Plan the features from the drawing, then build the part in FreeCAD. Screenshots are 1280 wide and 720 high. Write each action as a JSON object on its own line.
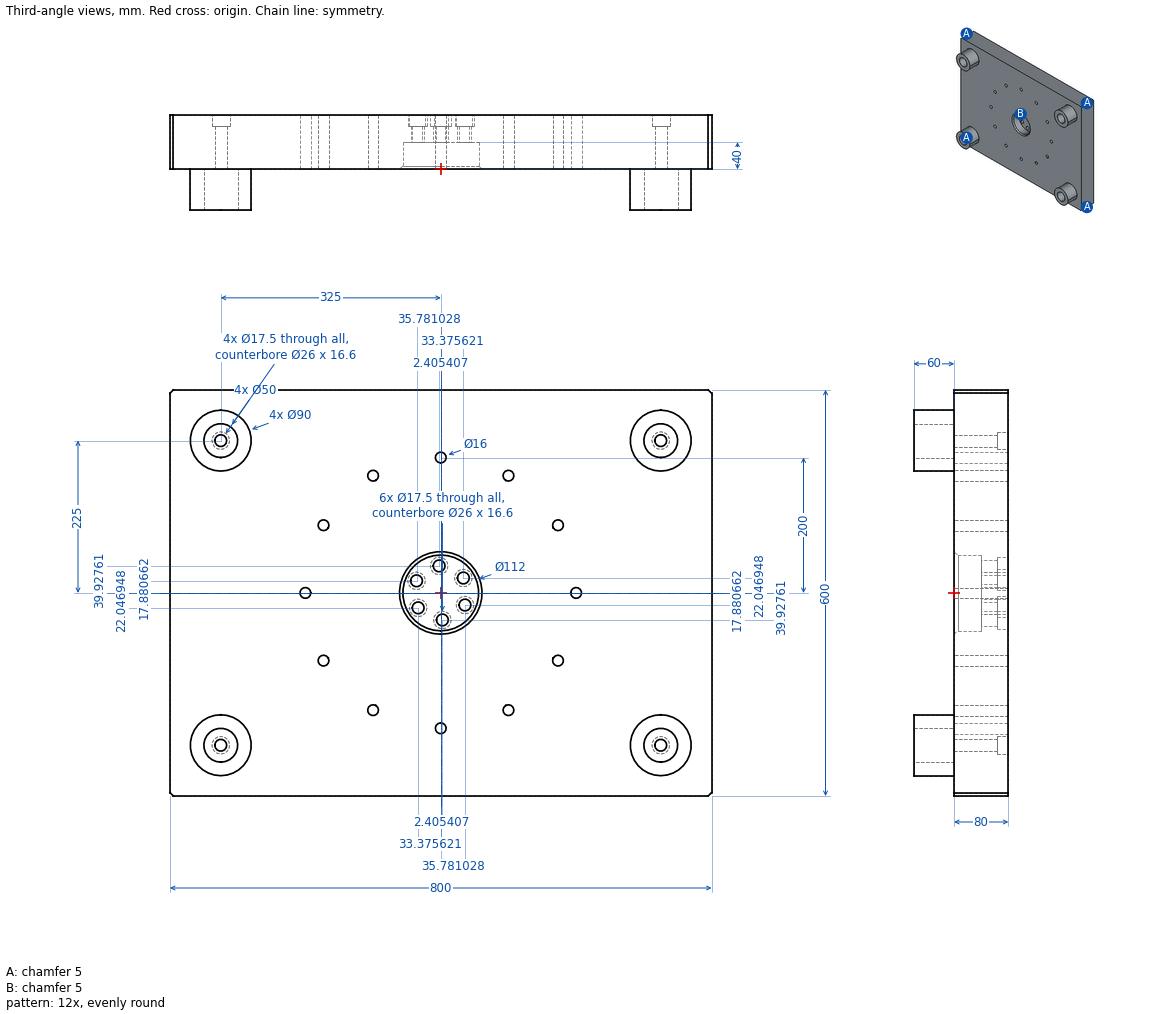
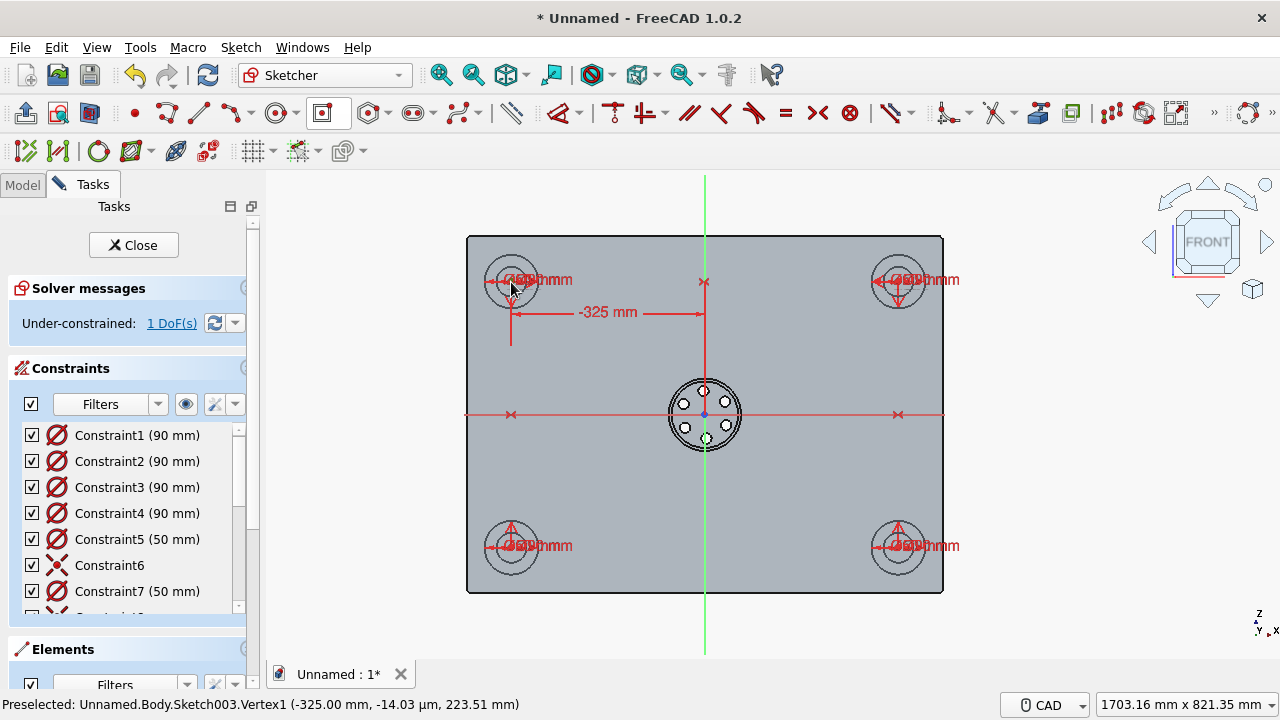
{"action": "key", "text": "i"}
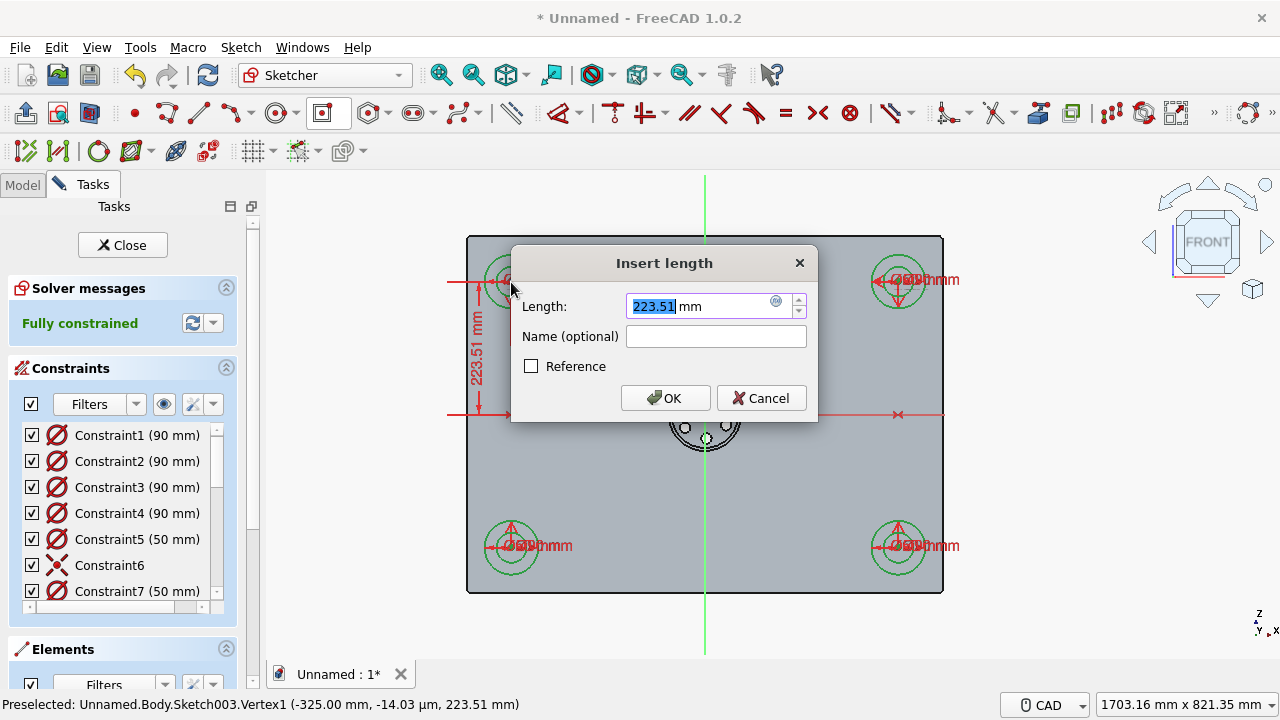
{"action": "type", "text": "225"}
{"action": "key", "text": "Return"}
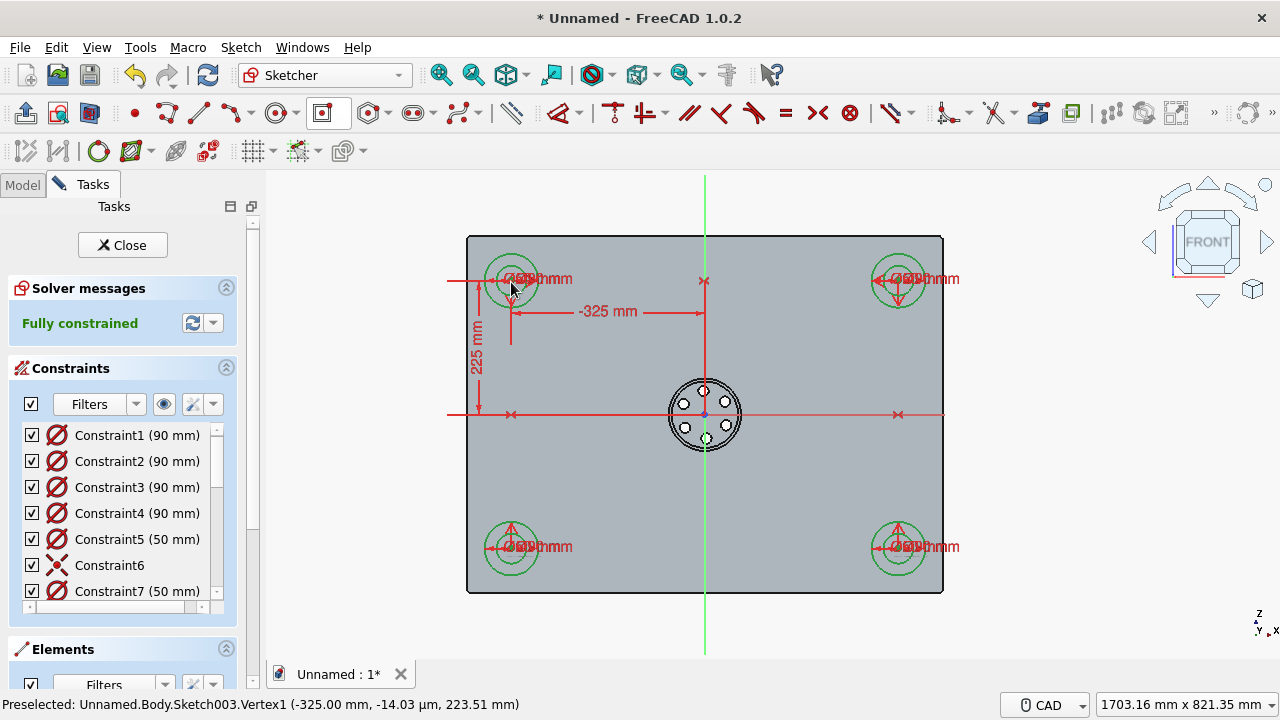
{"action": "left_click", "coordinate": [123, 245]}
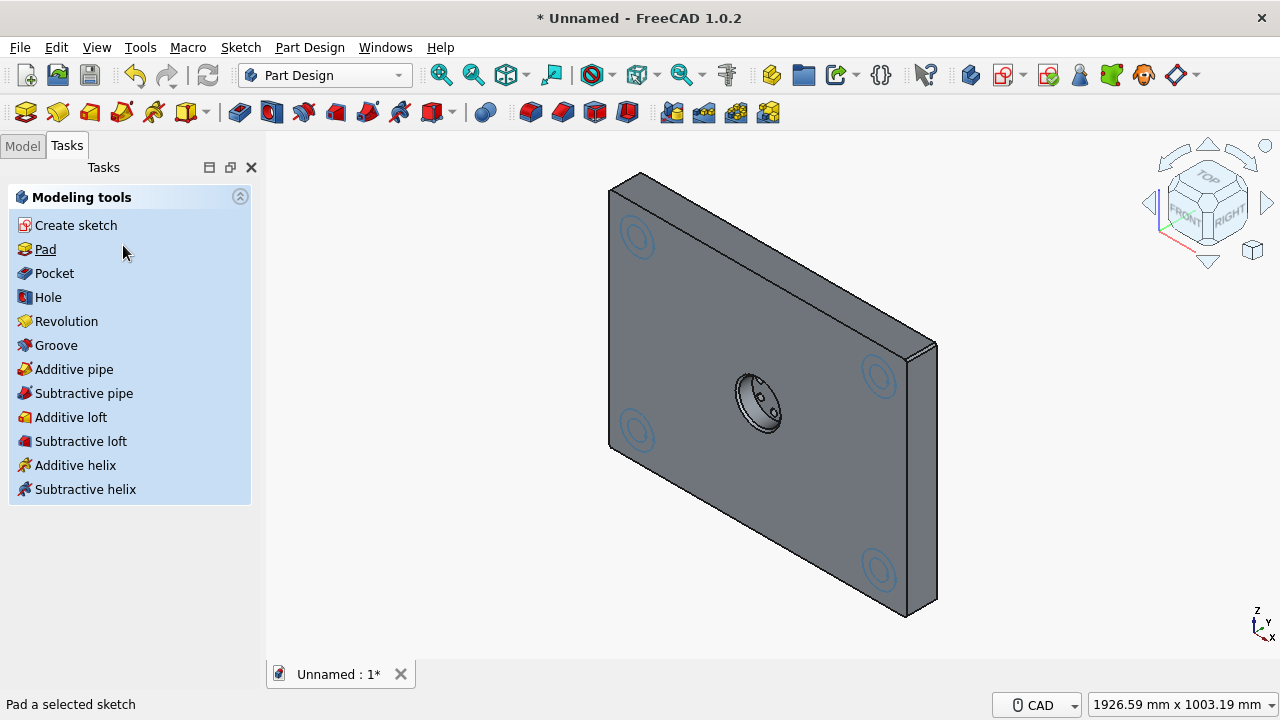
{"action": "left_click", "coordinate": [26, 112]}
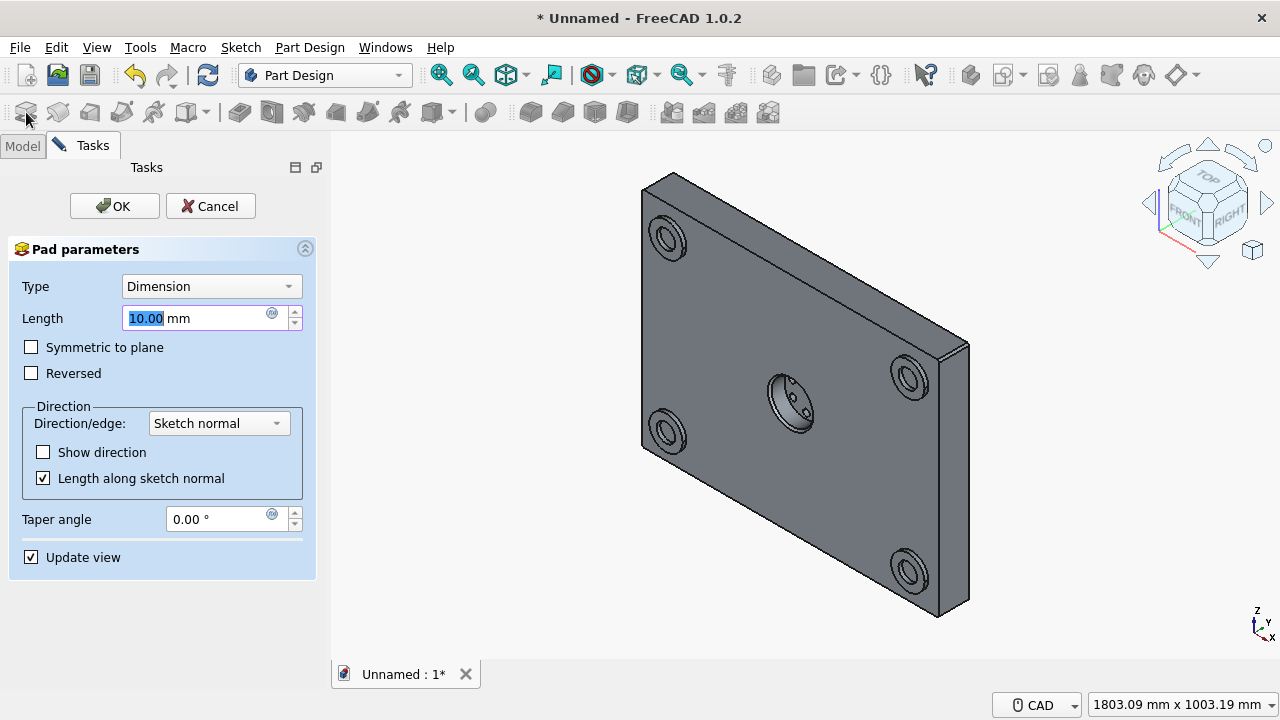
{"action": "type", "text": "60"}
{"action": "key", "text": "Tab"}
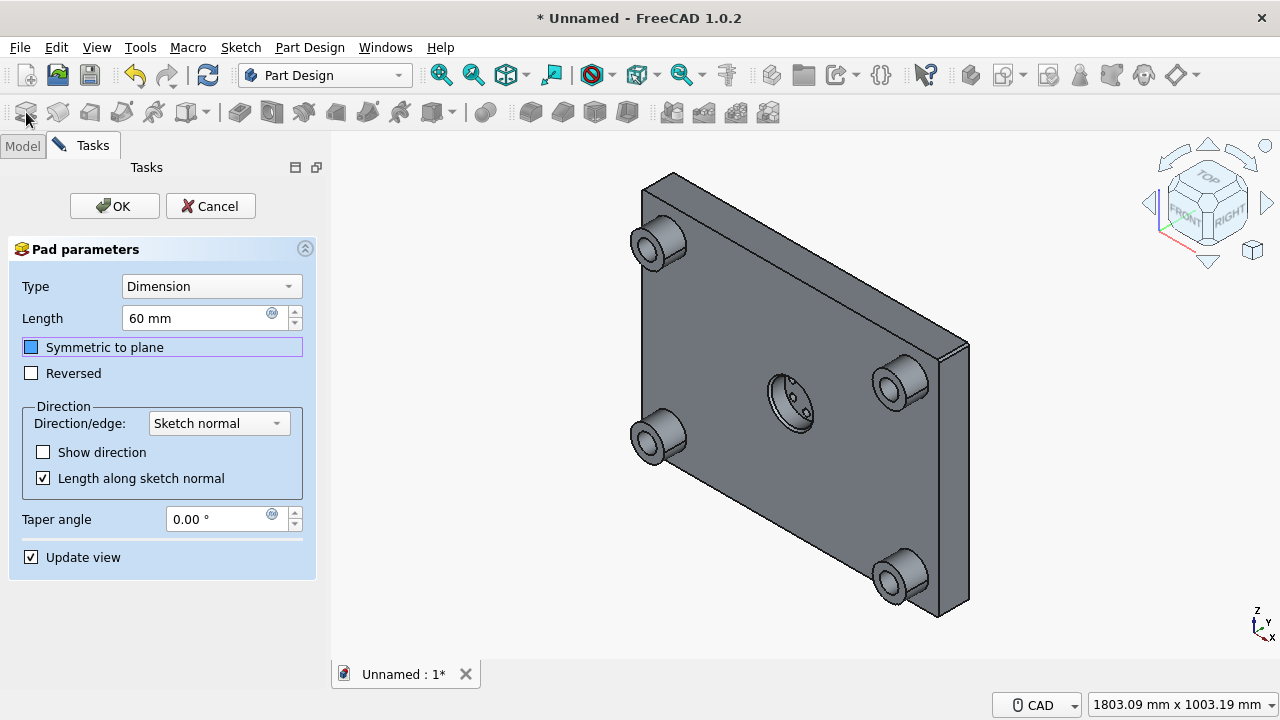
{"action": "left_click", "coordinate": [115, 206]}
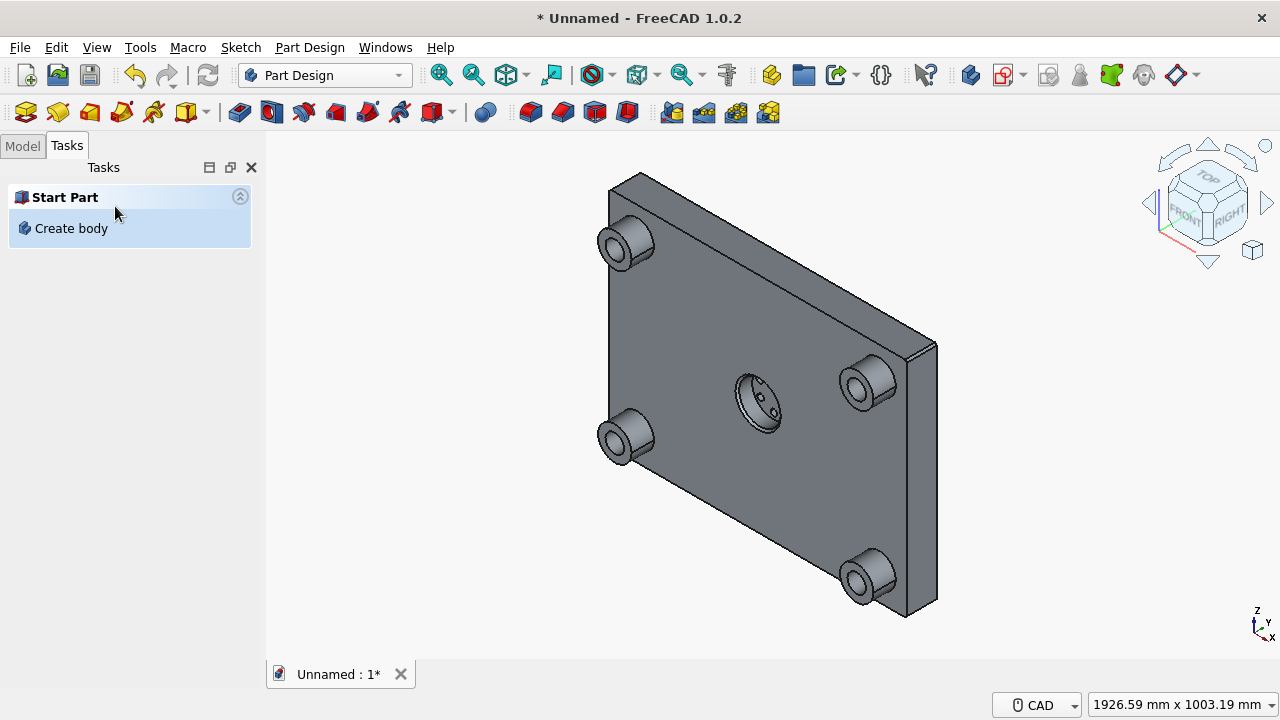
{"action": "key", "text": "4"}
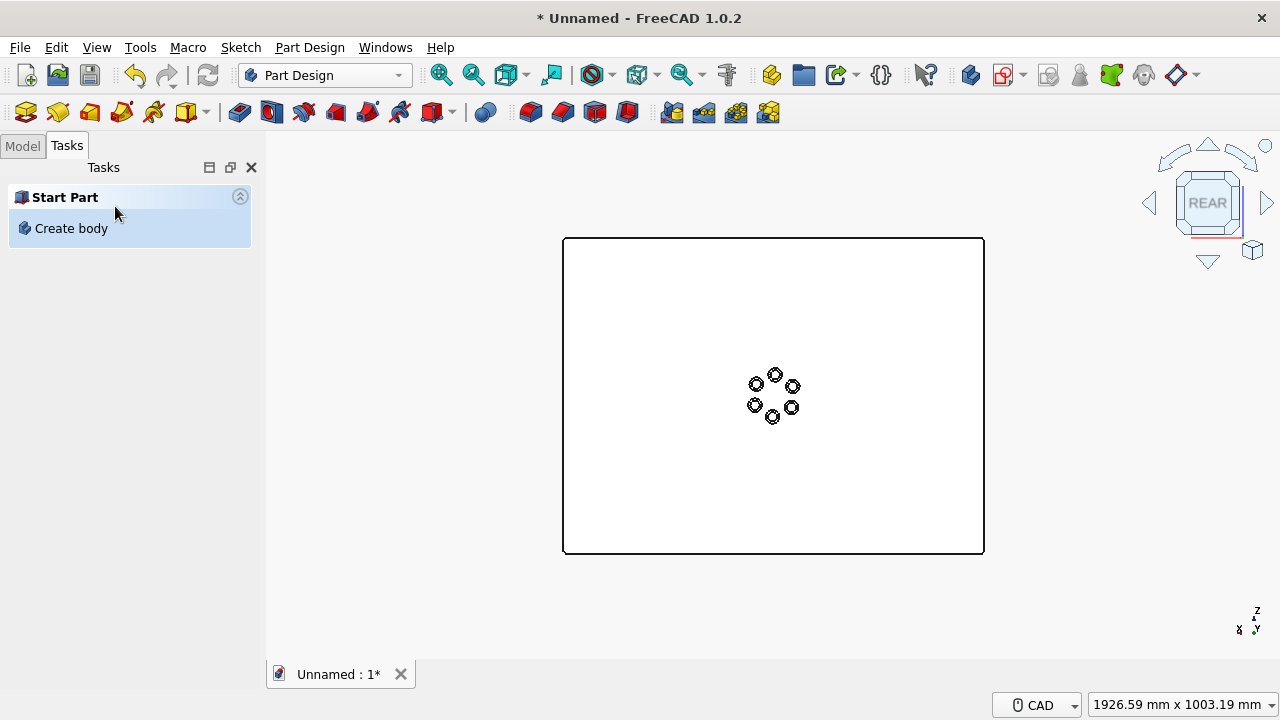
{"action": "left_click", "coordinate": [654, 350]}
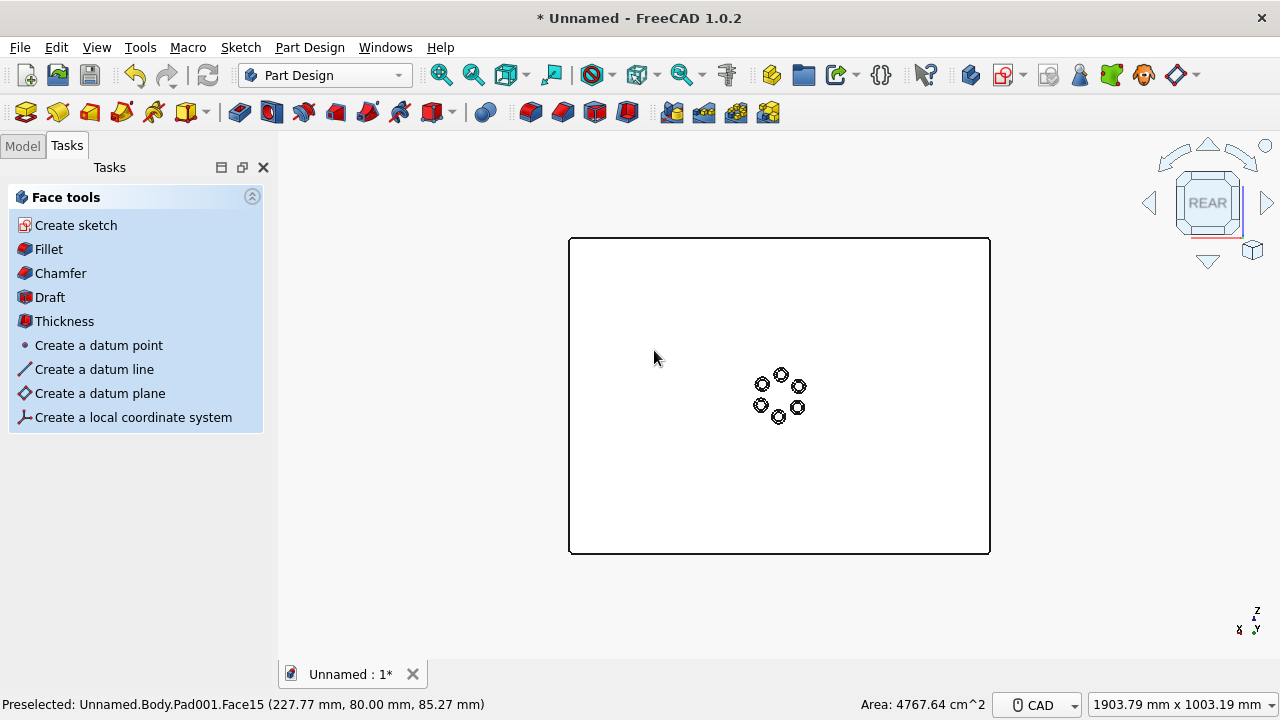
{"action": "left_click", "coordinate": [1004, 76]}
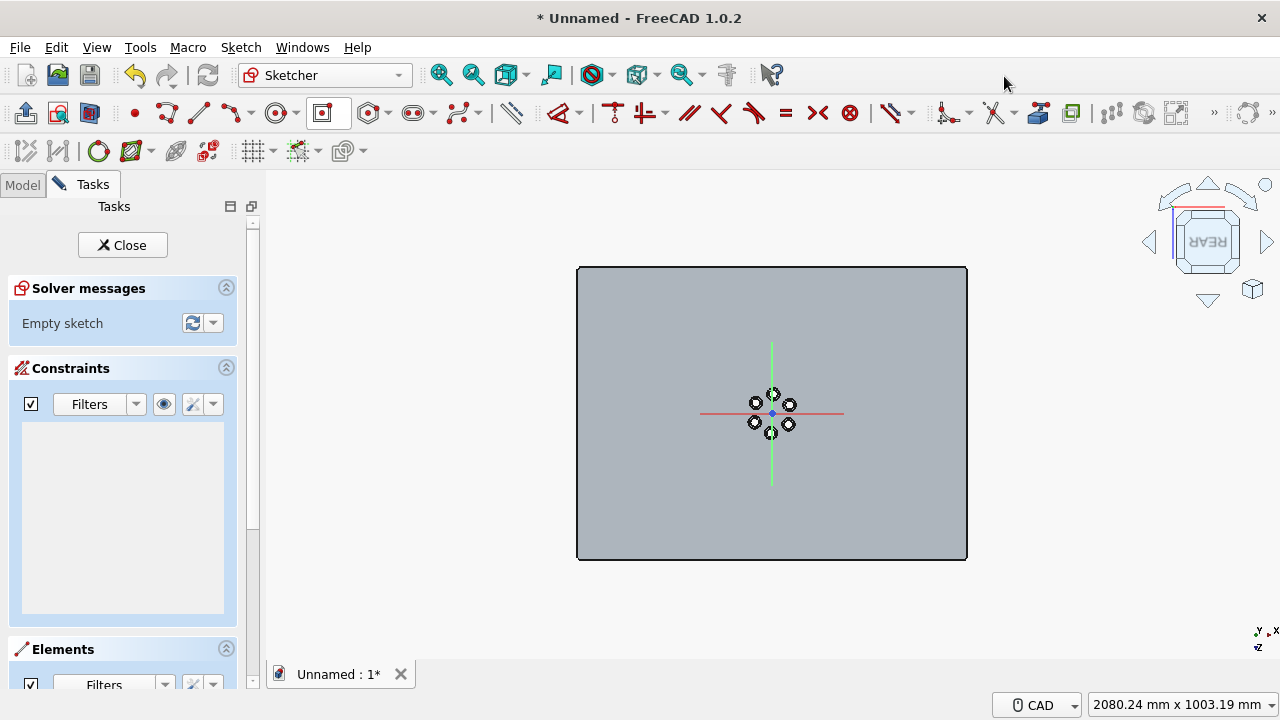
{"action": "key", "text": "g c"}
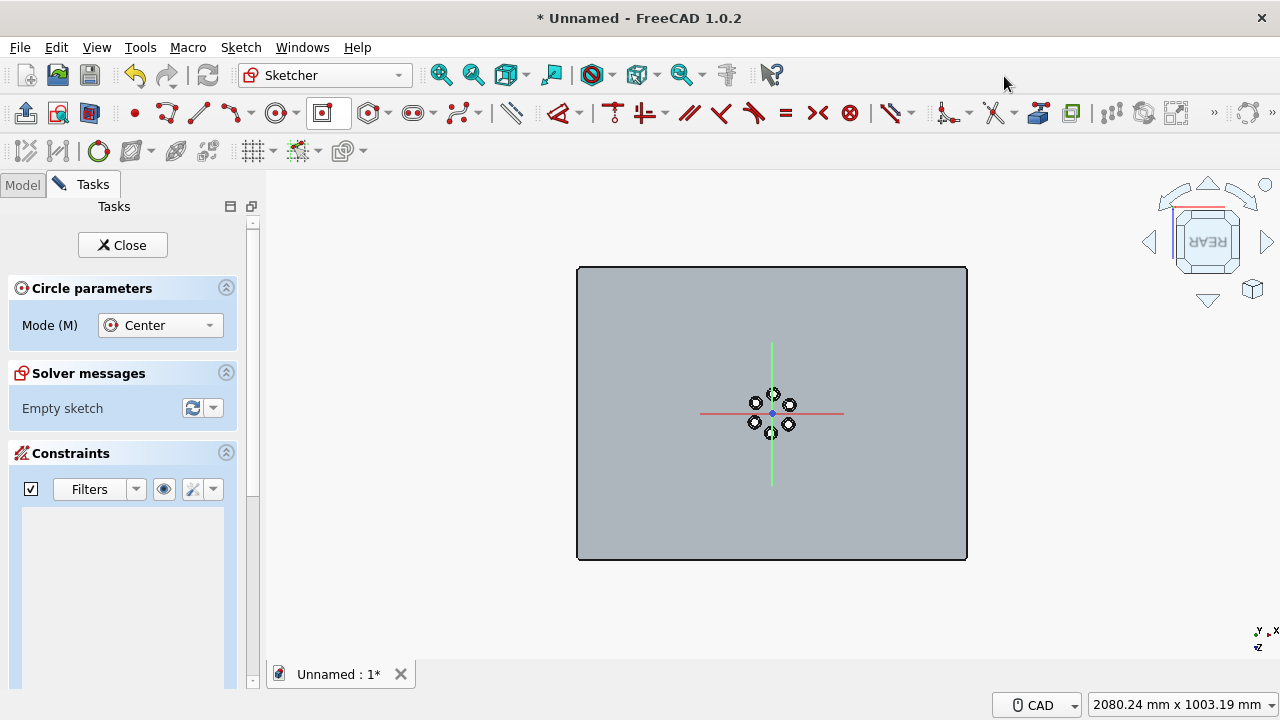
{"action": "scroll", "coordinate": [614, 523], "scroll_direction": "up", "scroll_amount": 9}